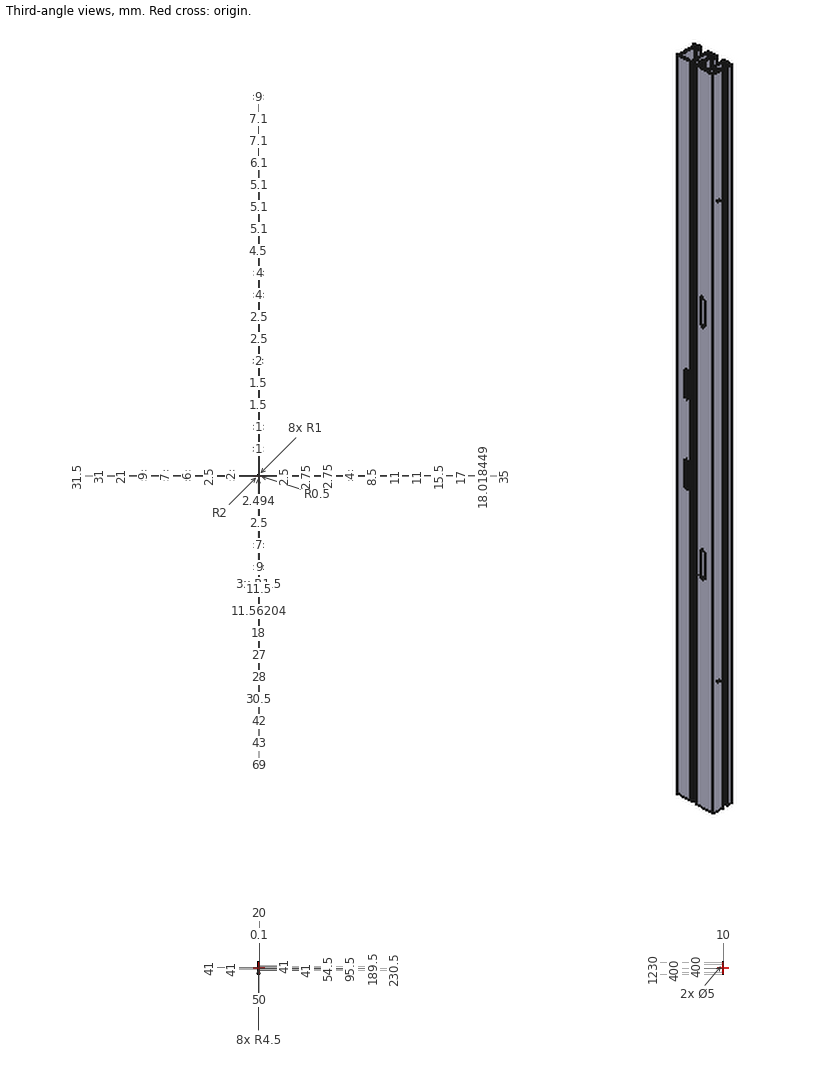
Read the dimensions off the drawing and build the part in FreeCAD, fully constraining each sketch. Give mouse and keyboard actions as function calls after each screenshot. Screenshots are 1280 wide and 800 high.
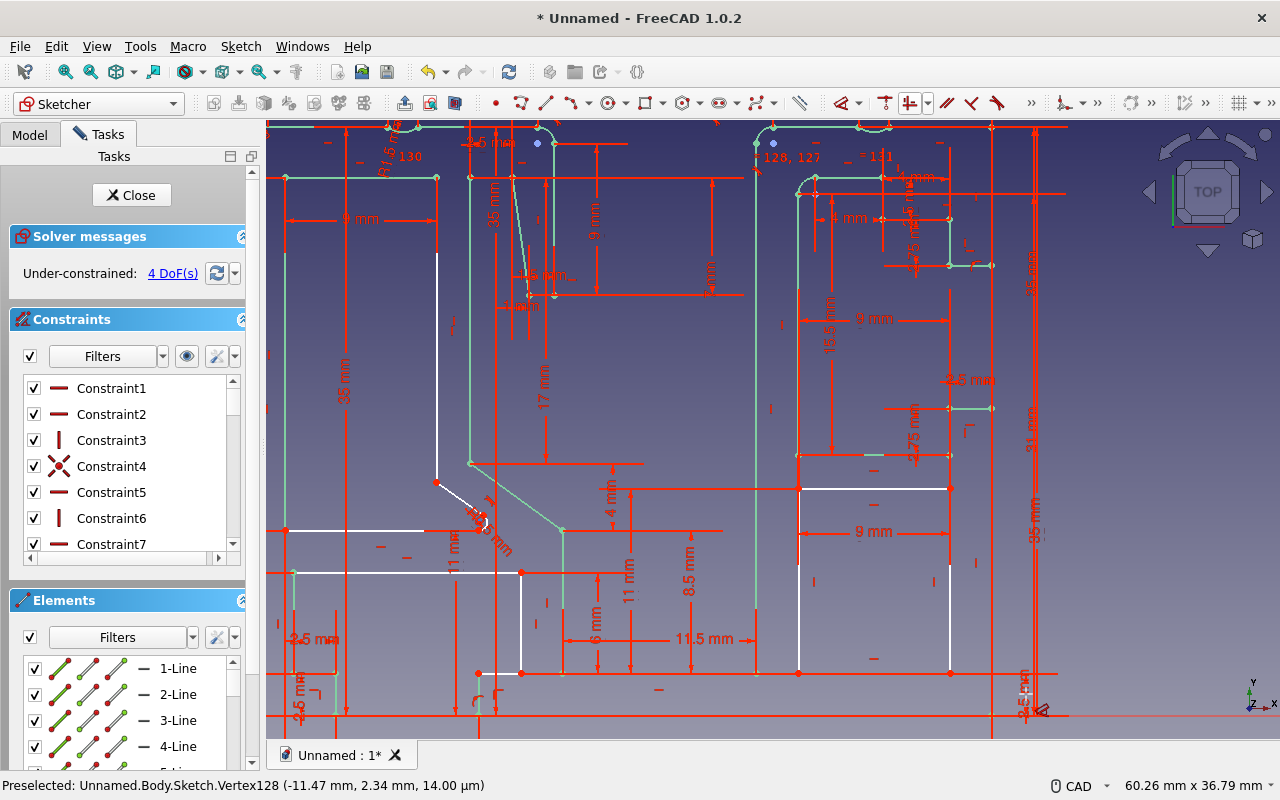
click(950, 674)
click(971, 640)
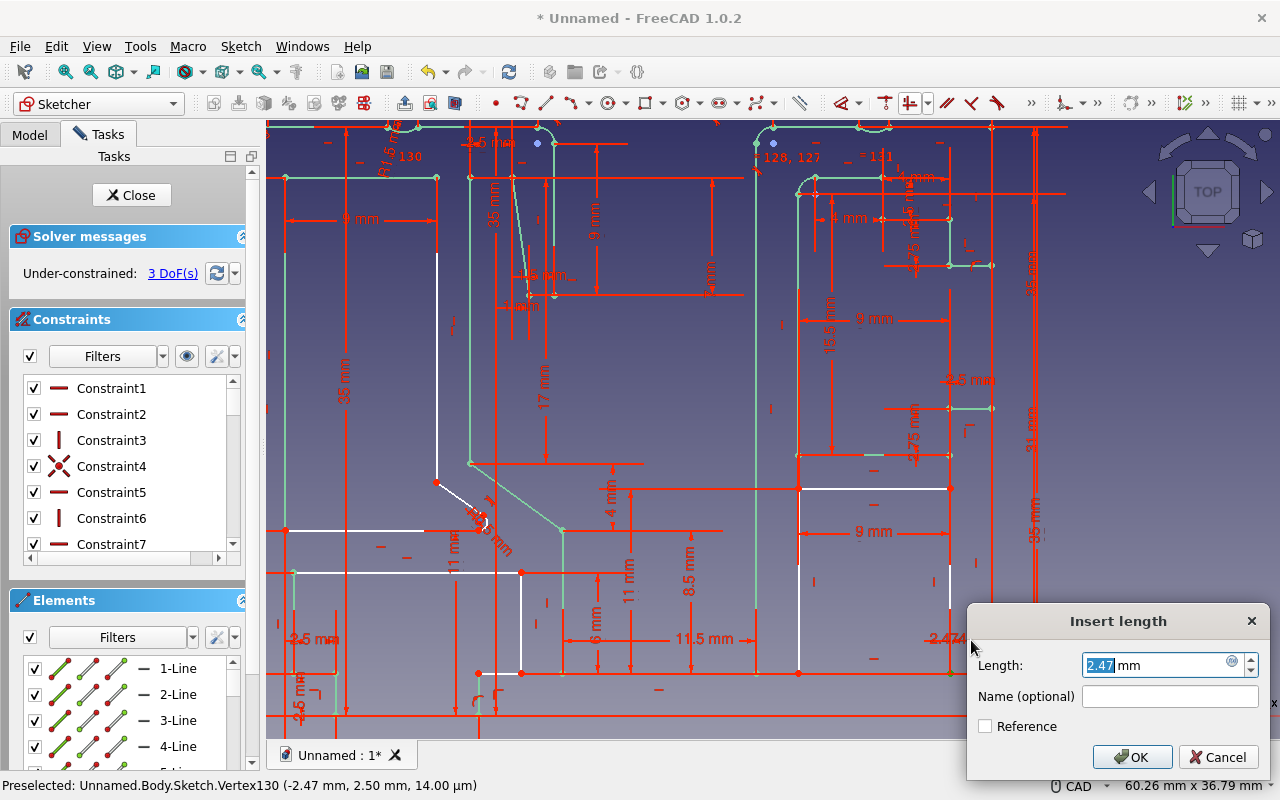
text(2.5)
key(Return)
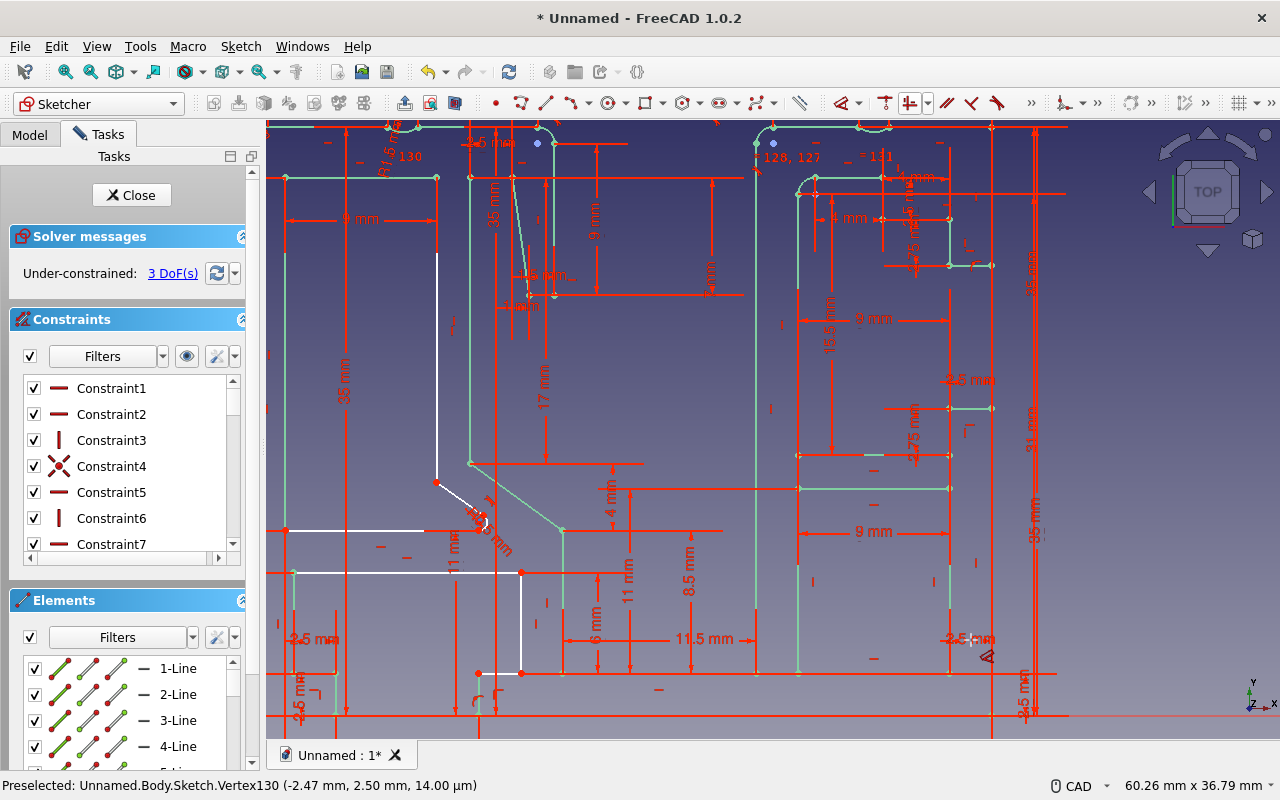
click(508, 674)
click(500, 640)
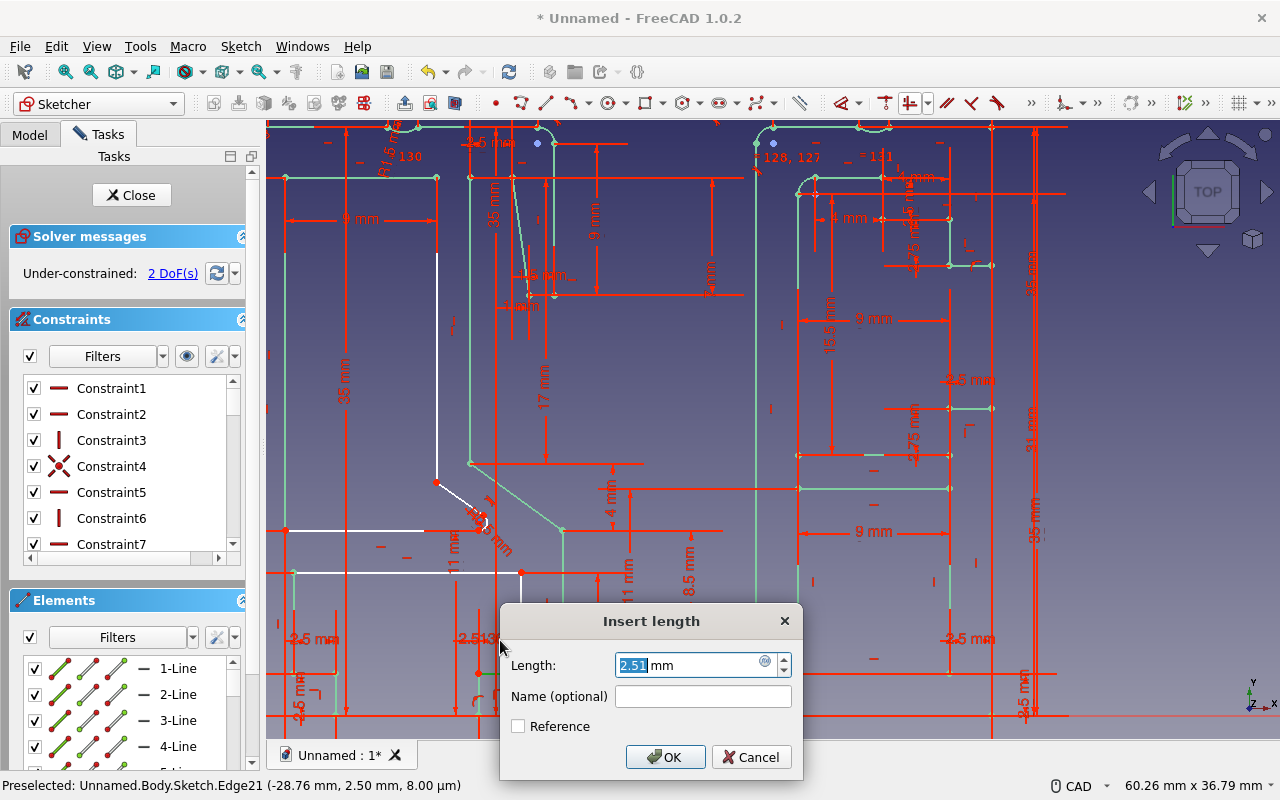
text(2.494)
key(Return)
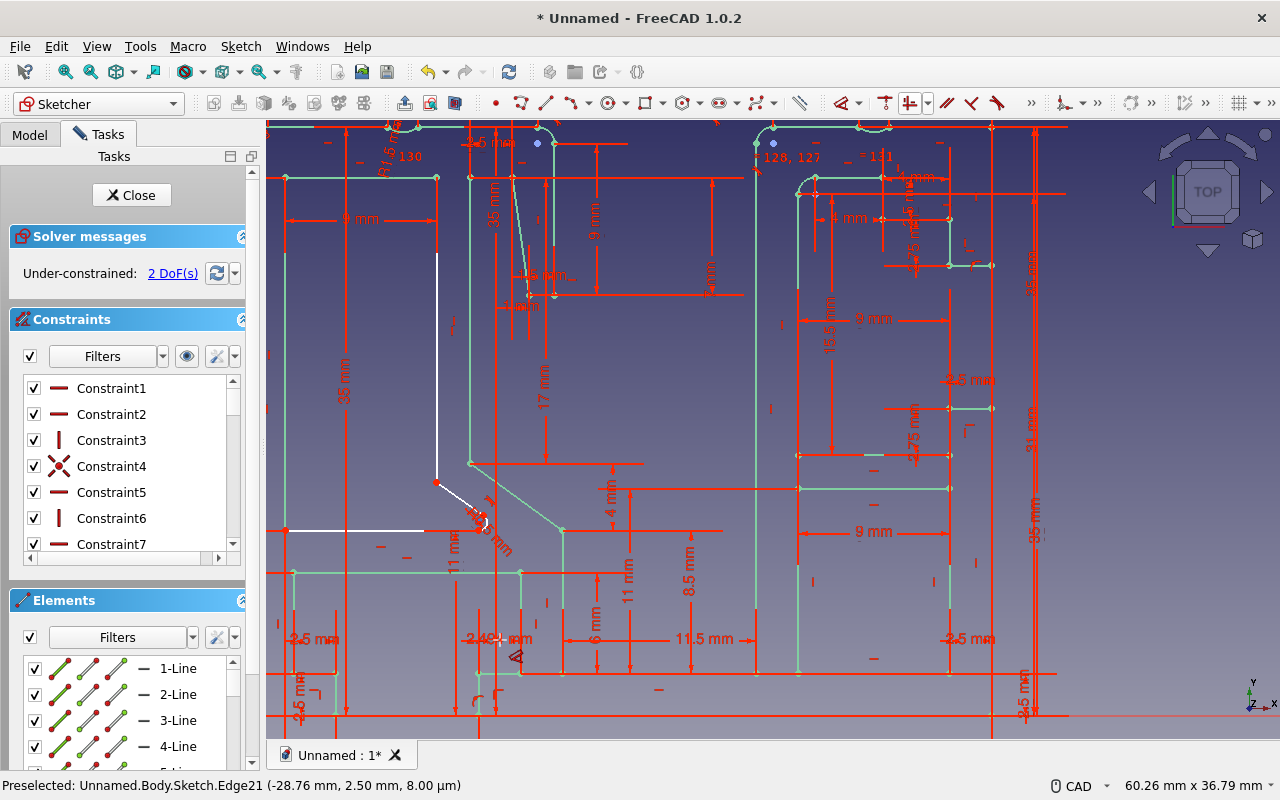
click(421, 531)
click(386, 497)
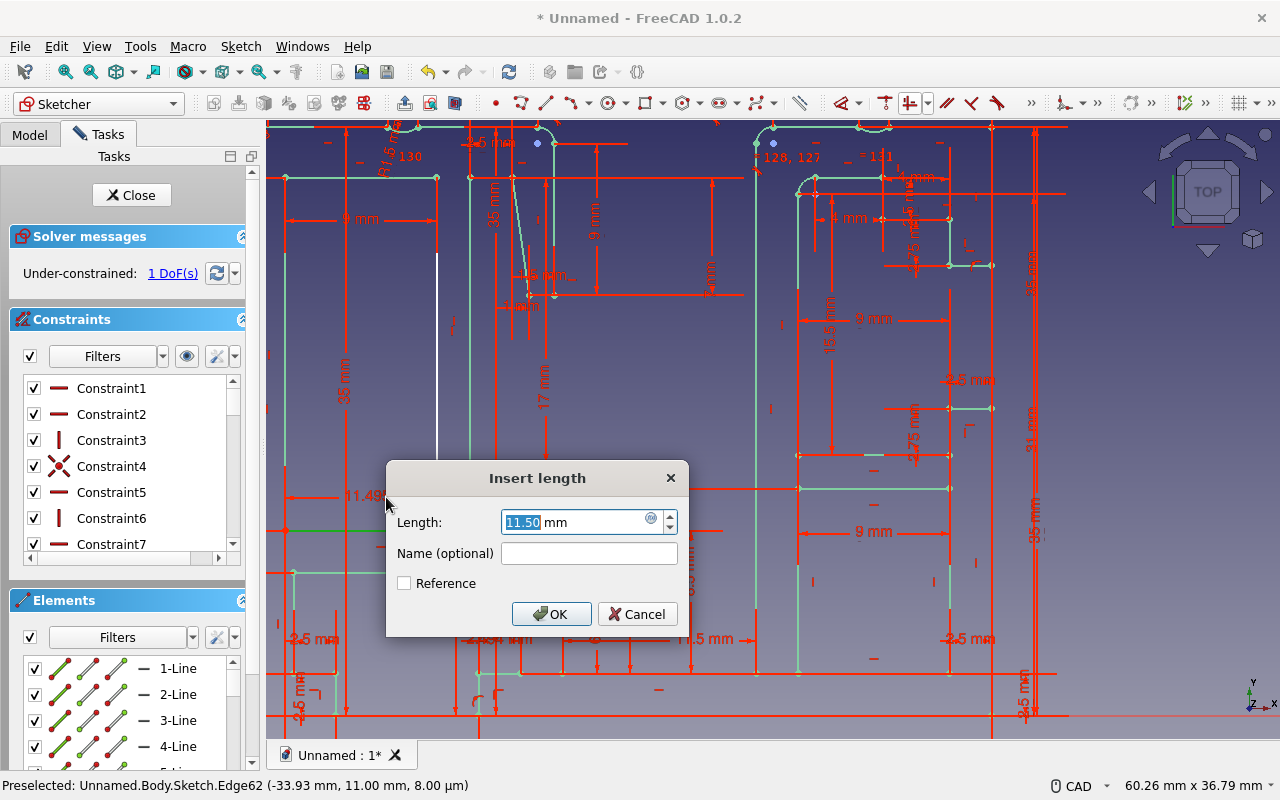
text(11.56204)
key(Return)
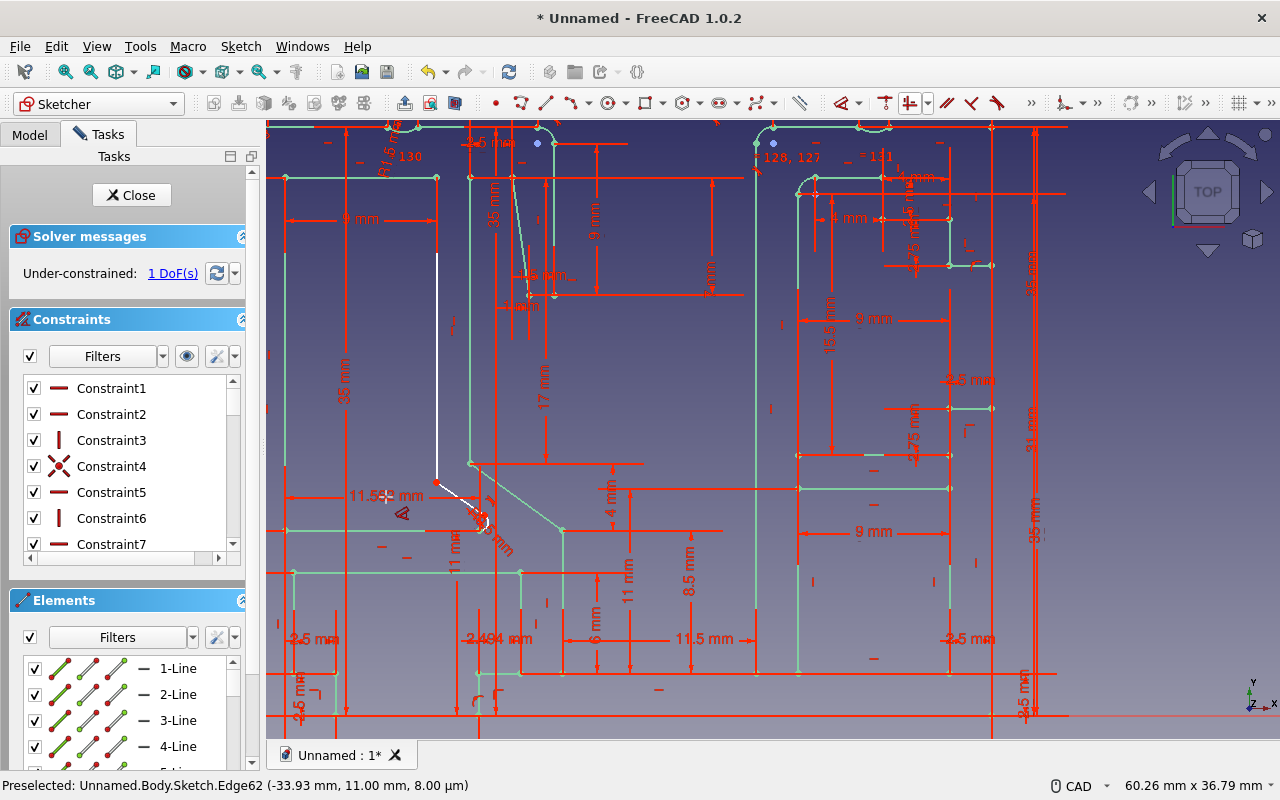
click(437, 269)
click(403, 330)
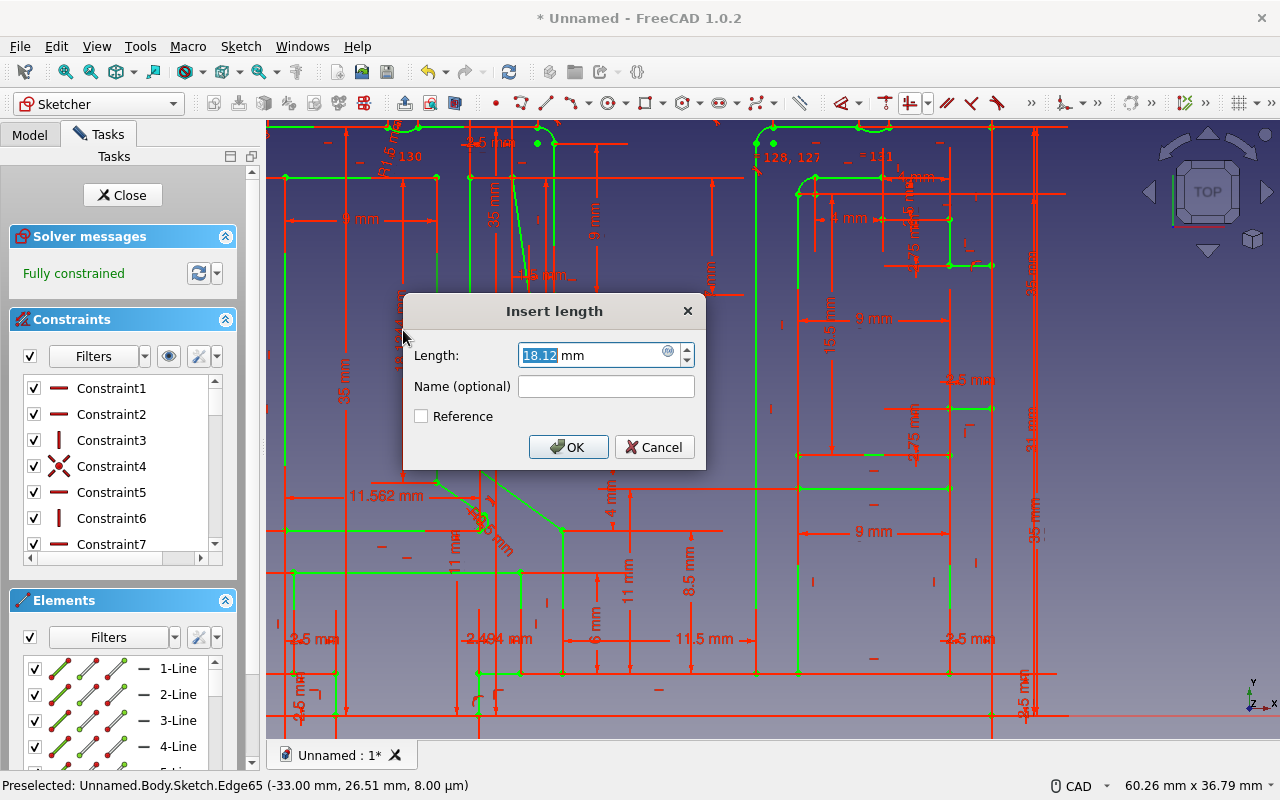
text(18.018449)
key(Return)
key(Escape)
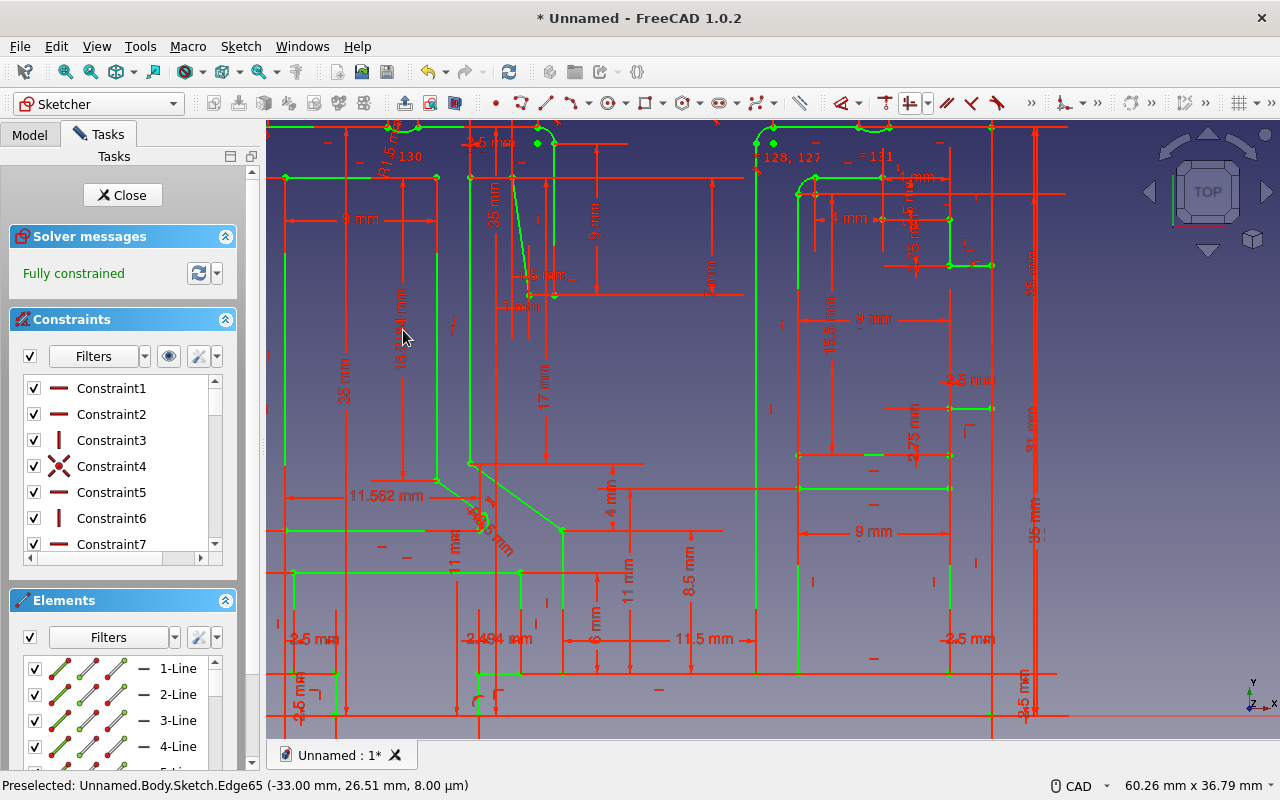
click(123, 195)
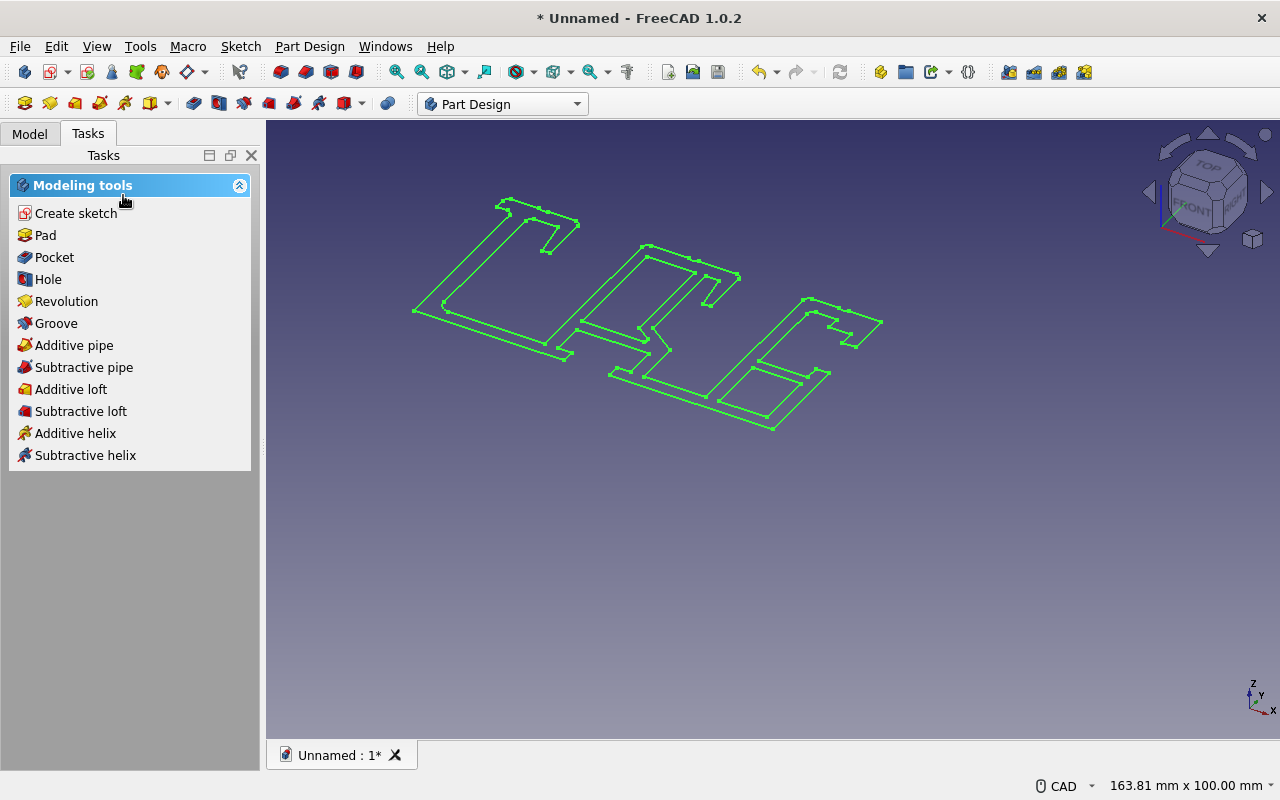
click(25, 104)